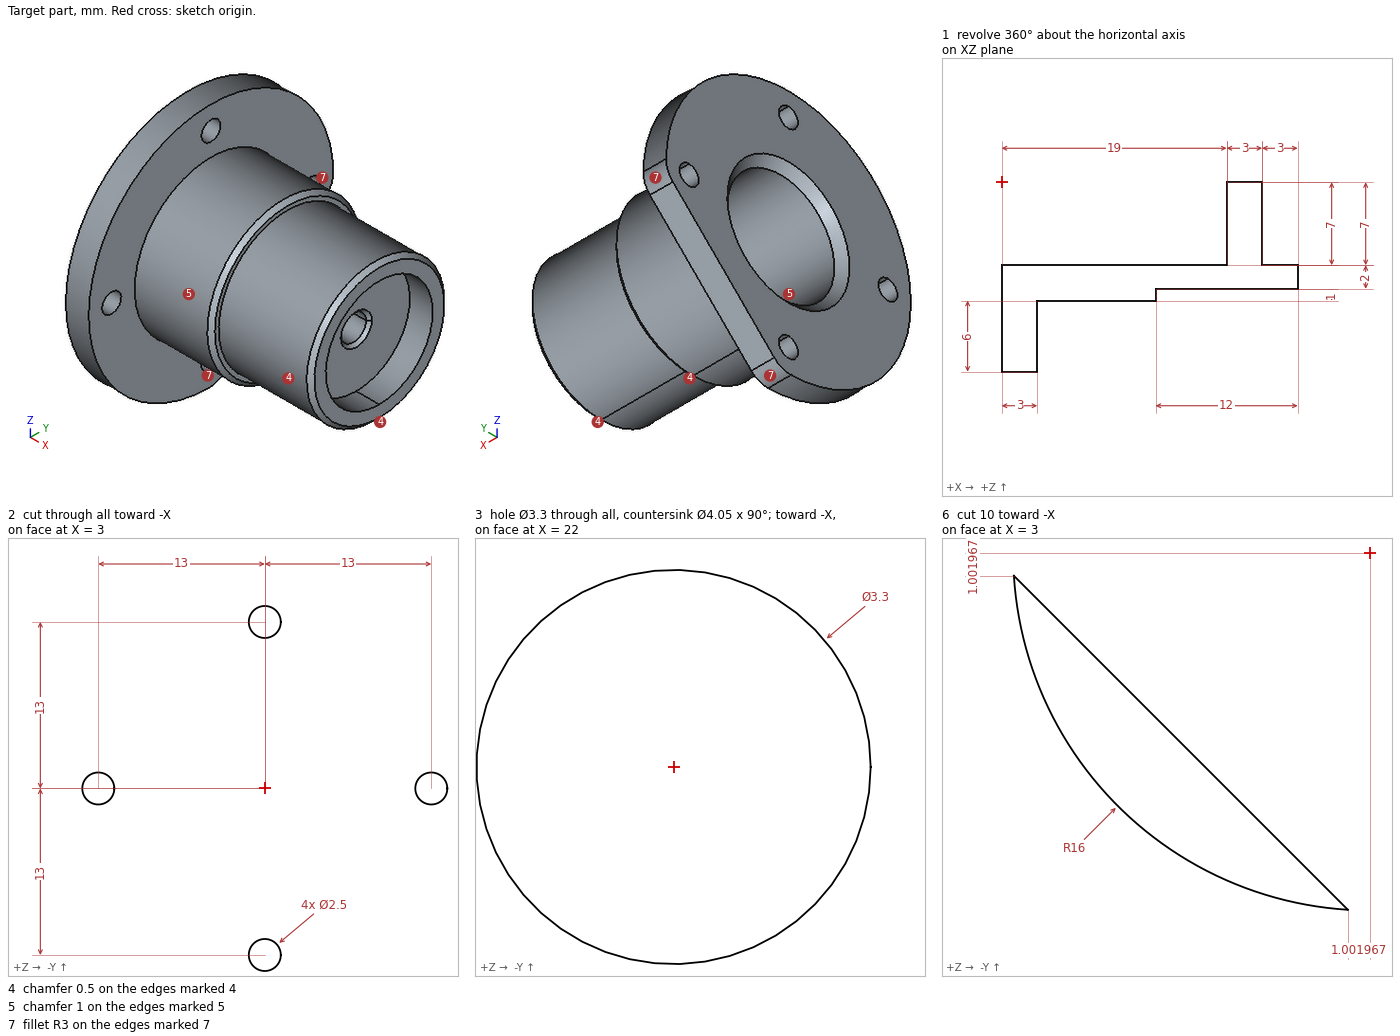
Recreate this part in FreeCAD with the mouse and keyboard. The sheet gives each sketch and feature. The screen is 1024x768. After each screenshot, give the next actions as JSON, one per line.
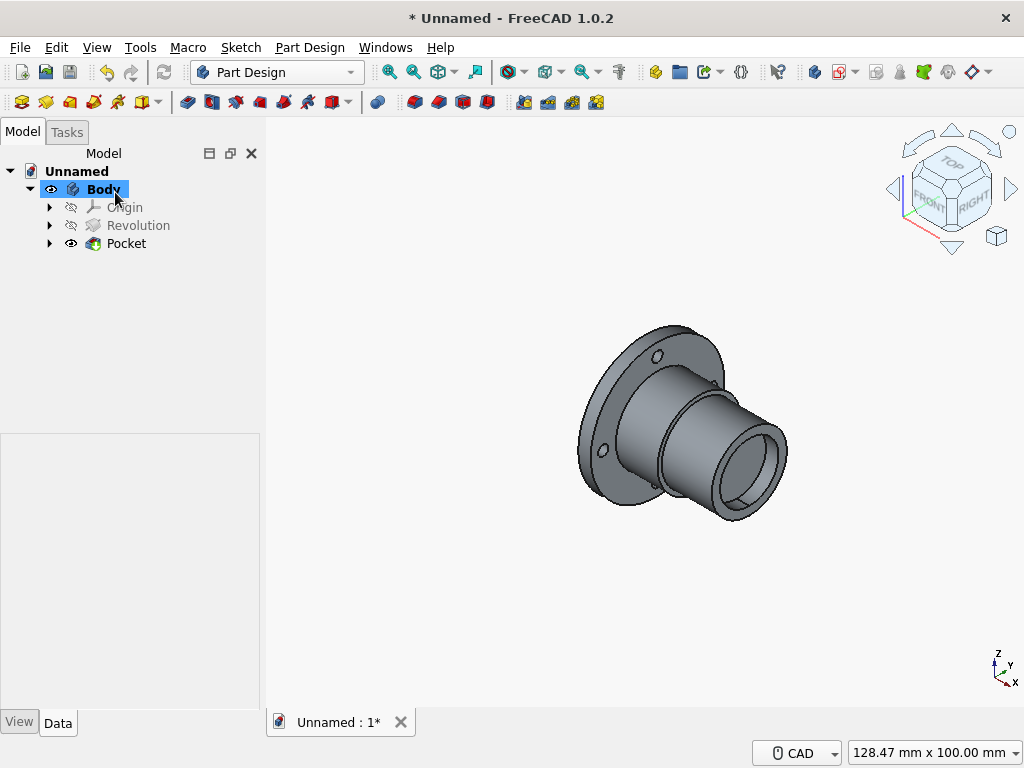
{"action": "left_click", "coordinate": [737, 464]}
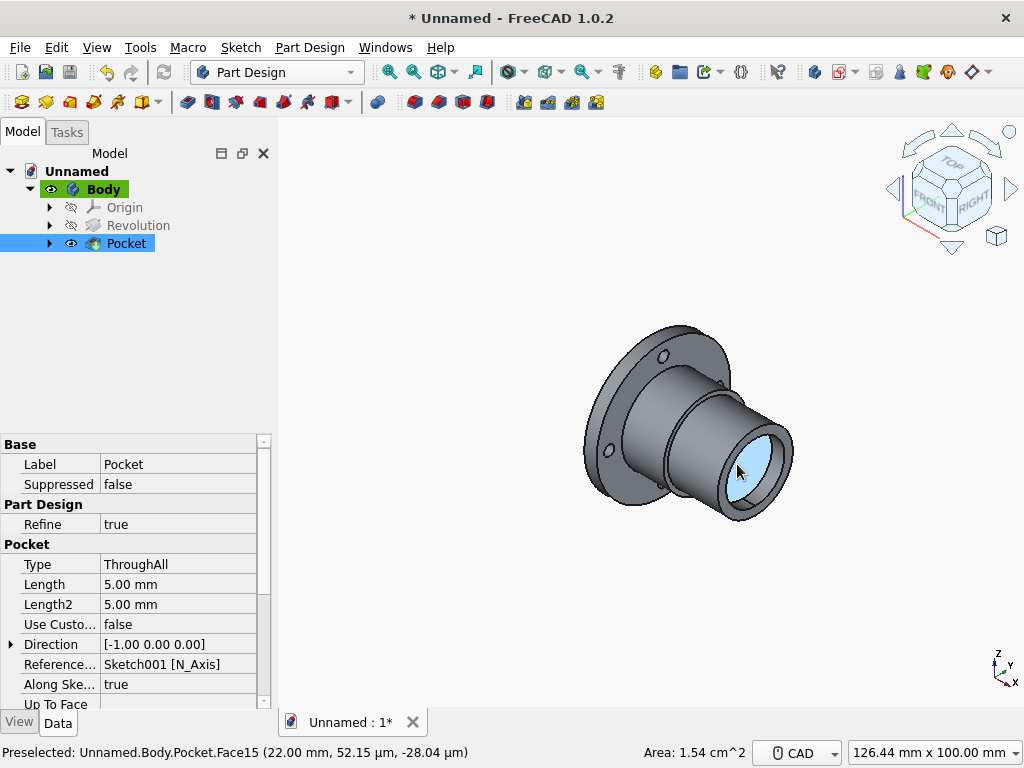
{"action": "left_click", "coordinate": [840, 72]}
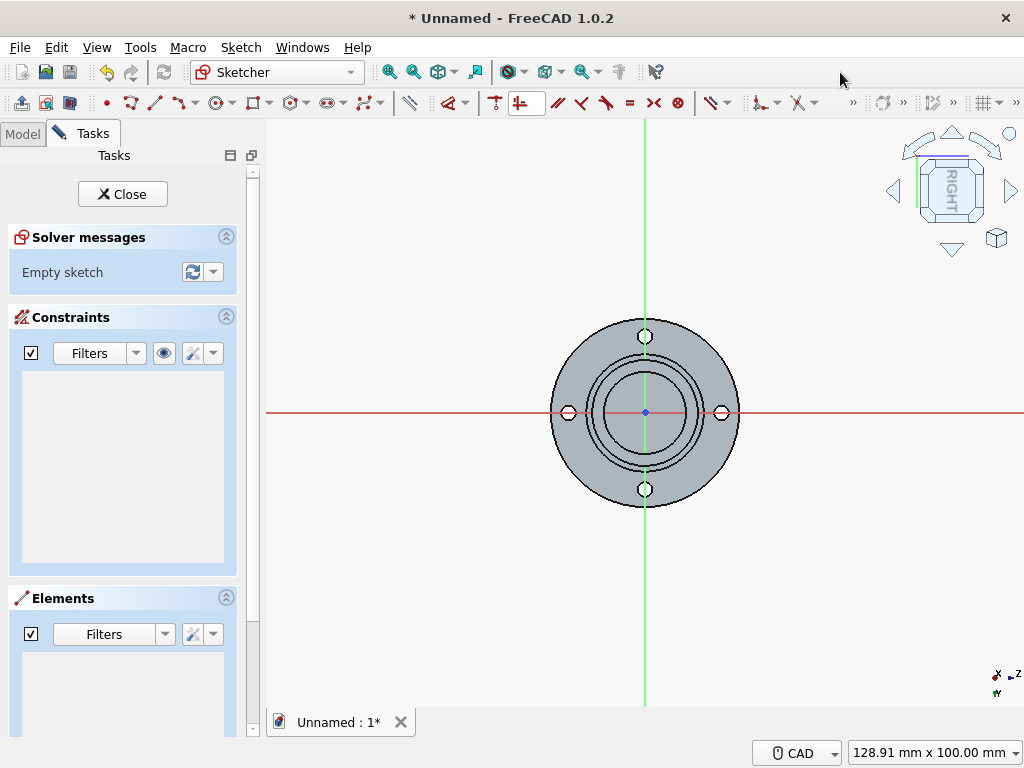
{"action": "scroll", "coordinate": [649, 413], "scroll_direction": "up", "scroll_amount": 15}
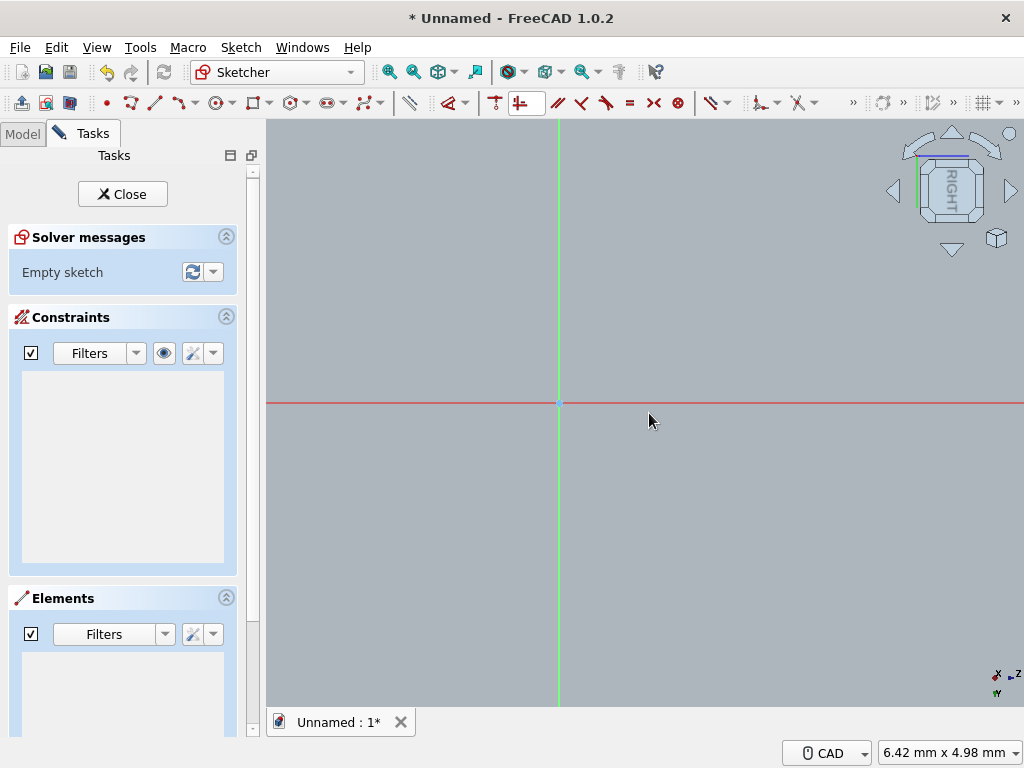
{"action": "left_click", "coordinate": [216, 104]}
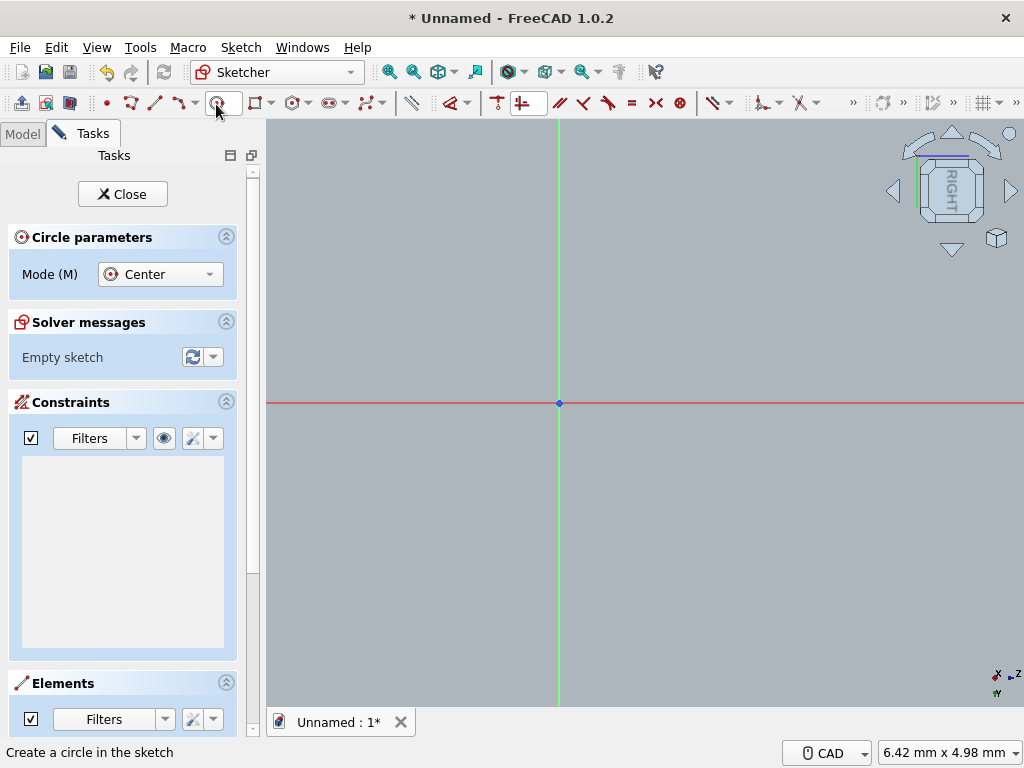
{"action": "left_click", "coordinate": [559, 403]}
{"action": "mouse_move", "coordinate": [697, 266]}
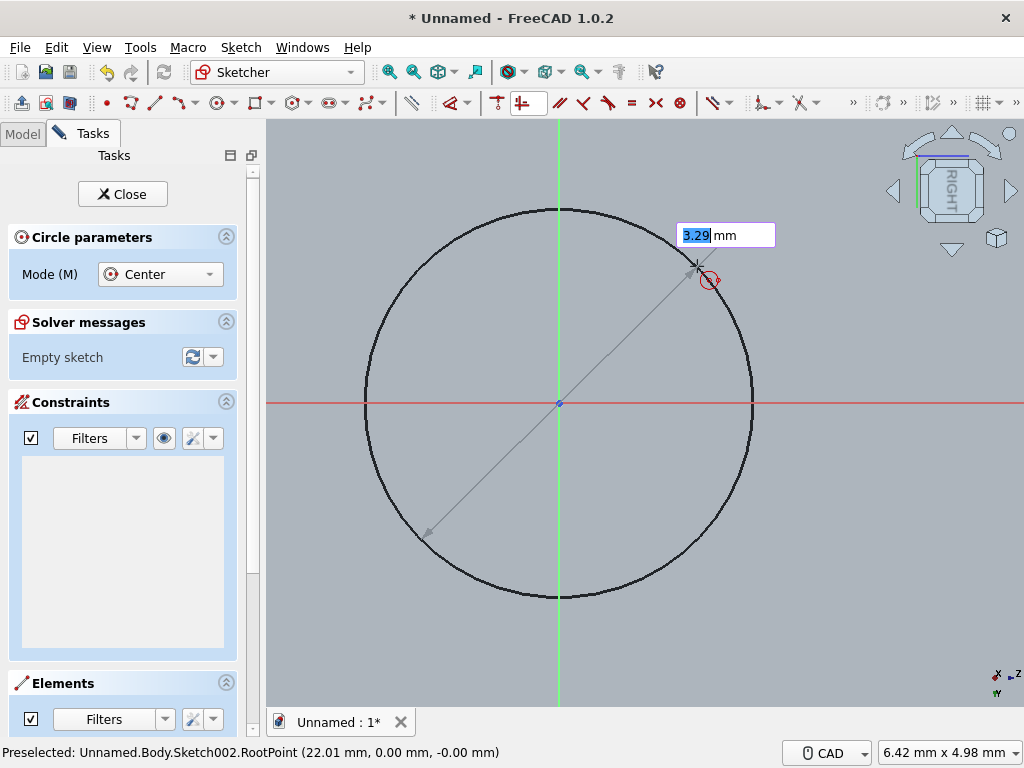
{"action": "type", "text": "3.3"}
{"action": "key", "text": "Return"}
{"action": "key", "text": "Escape"}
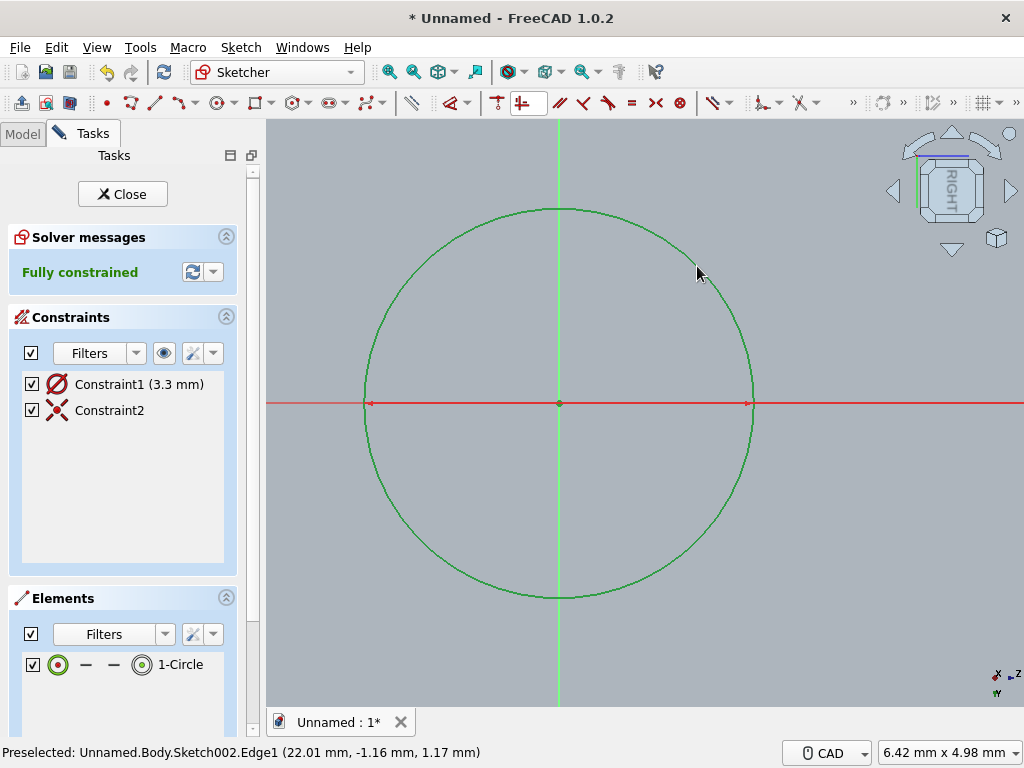
{"action": "left_click", "coordinate": [123, 194]}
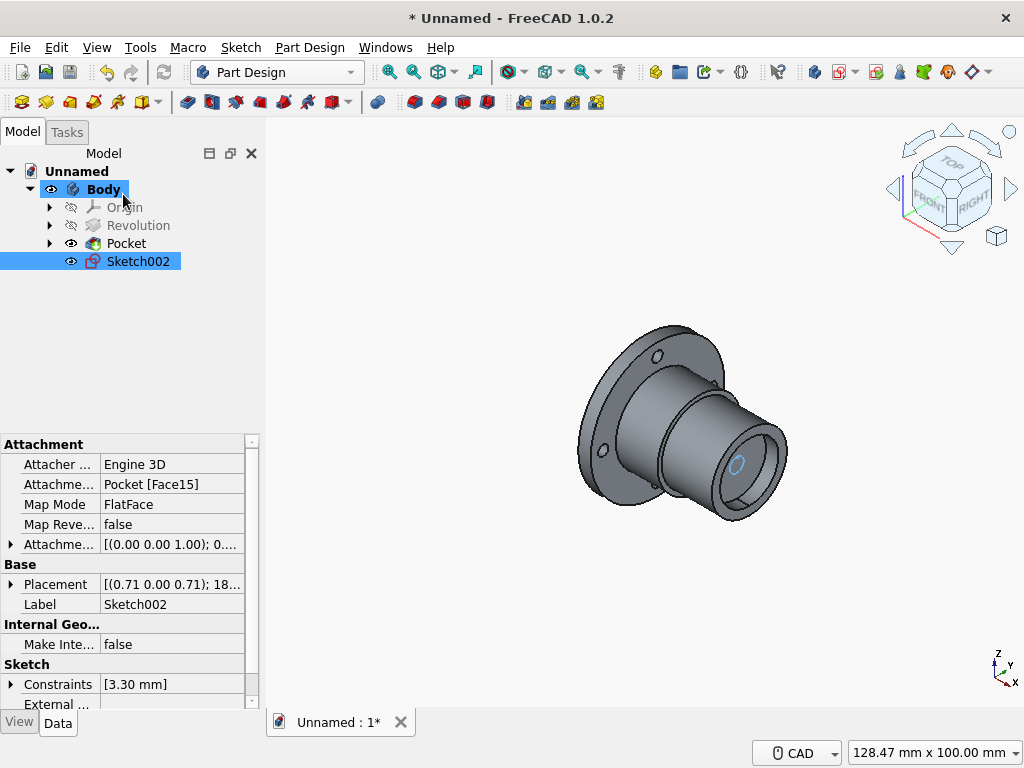
{"action": "left_click", "coordinate": [212, 102]}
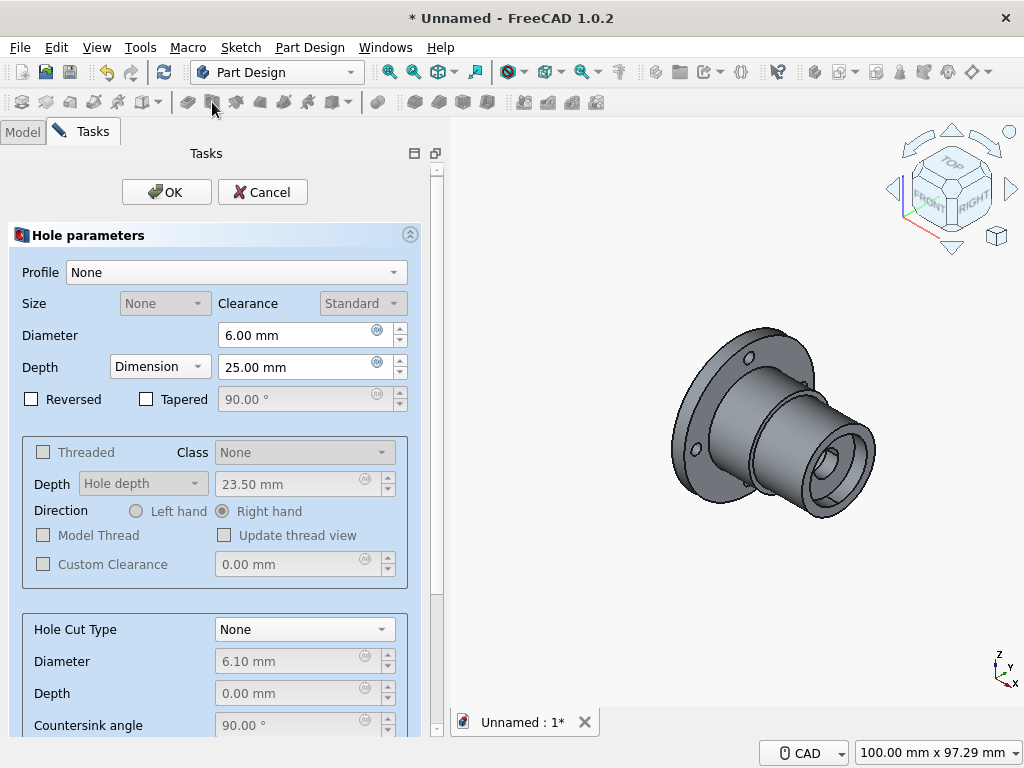
{"action": "triple_click", "coordinate": [305, 335]}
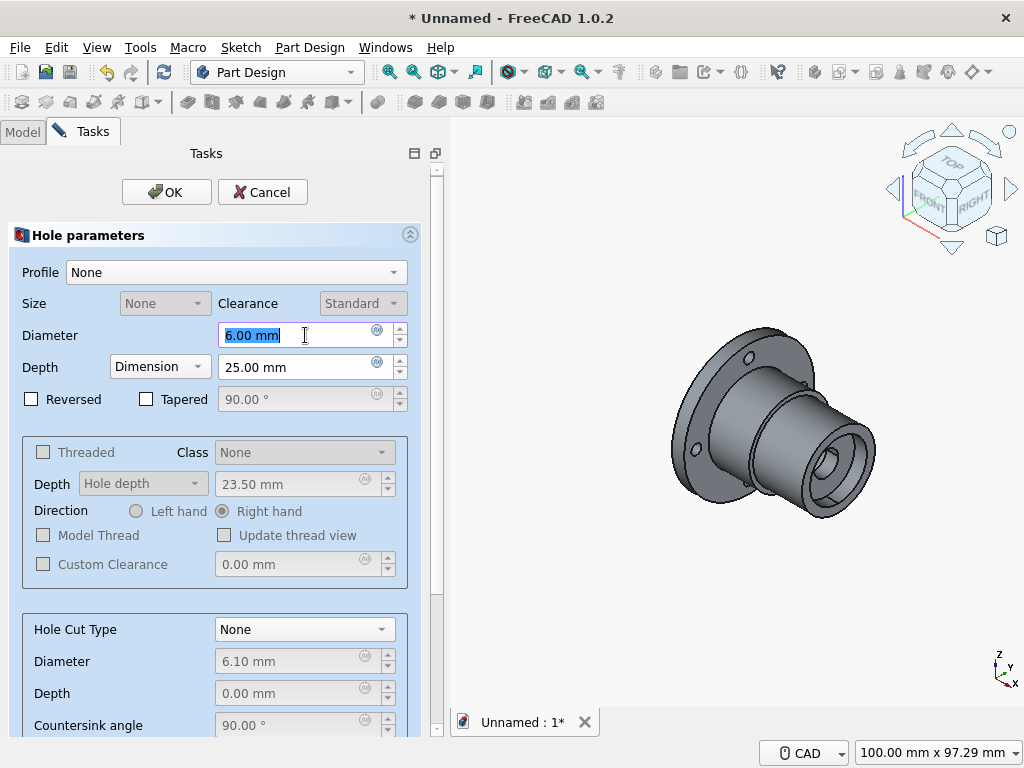
{"action": "type", "text": "3.3"}
{"action": "key", "text": "Tab"}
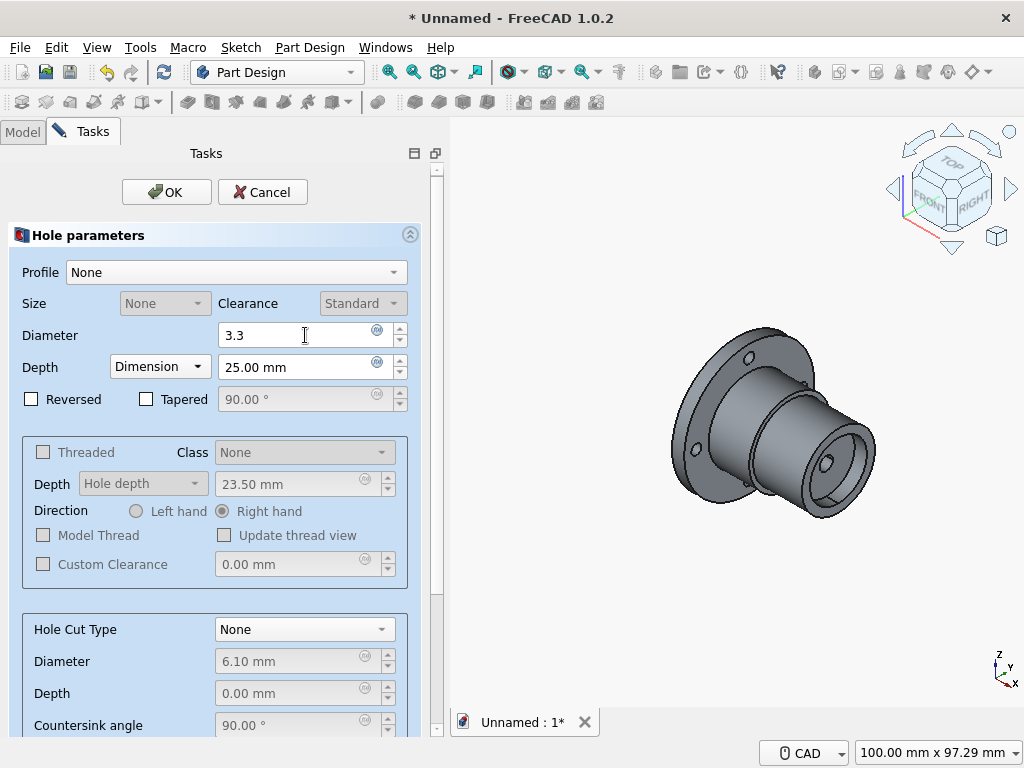
{"action": "left_click", "coordinate": [161, 366]}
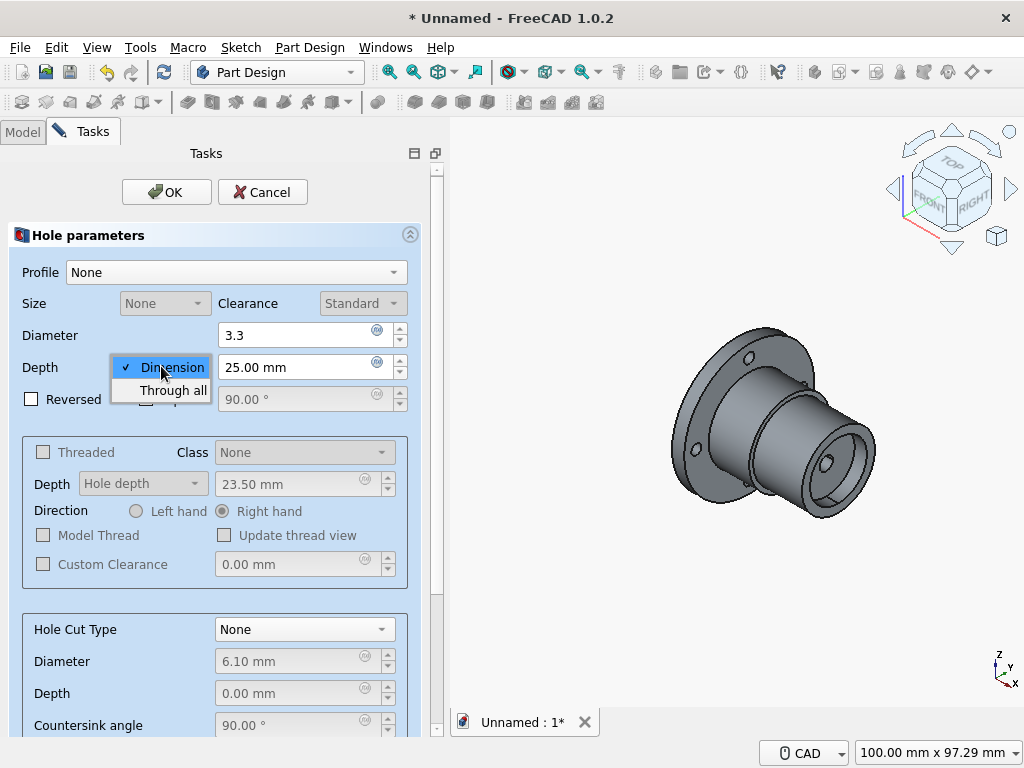
{"action": "left_click", "coordinate": [160, 390]}